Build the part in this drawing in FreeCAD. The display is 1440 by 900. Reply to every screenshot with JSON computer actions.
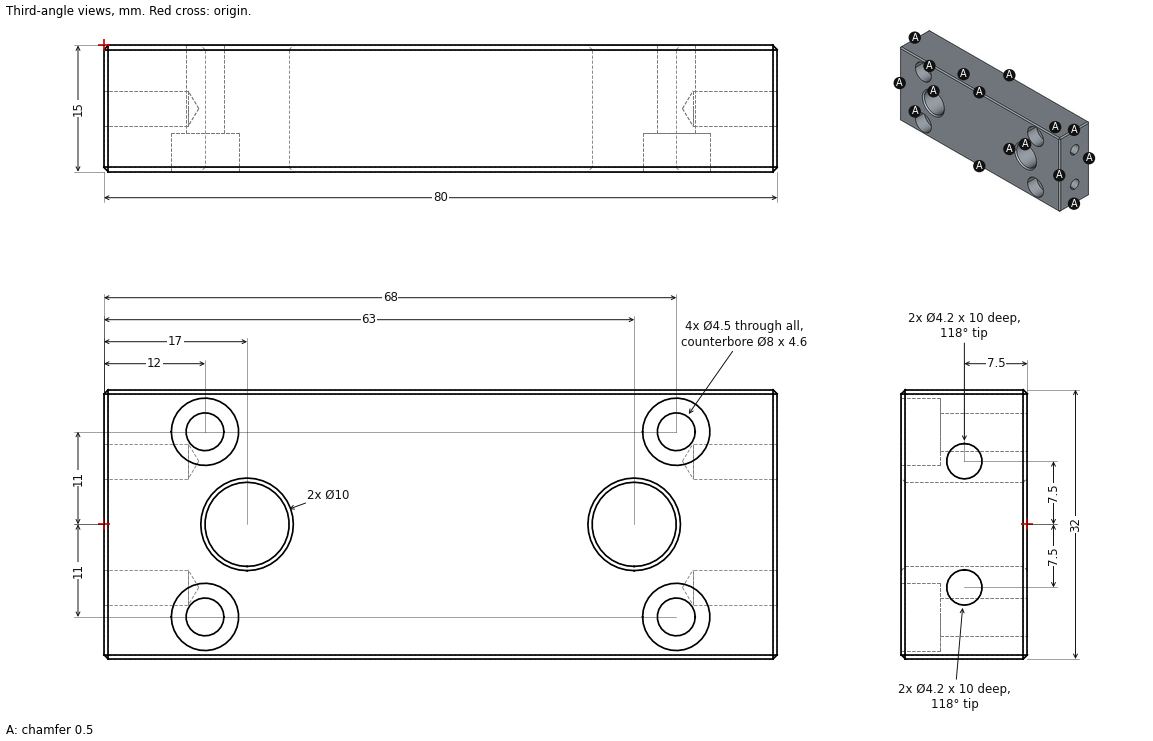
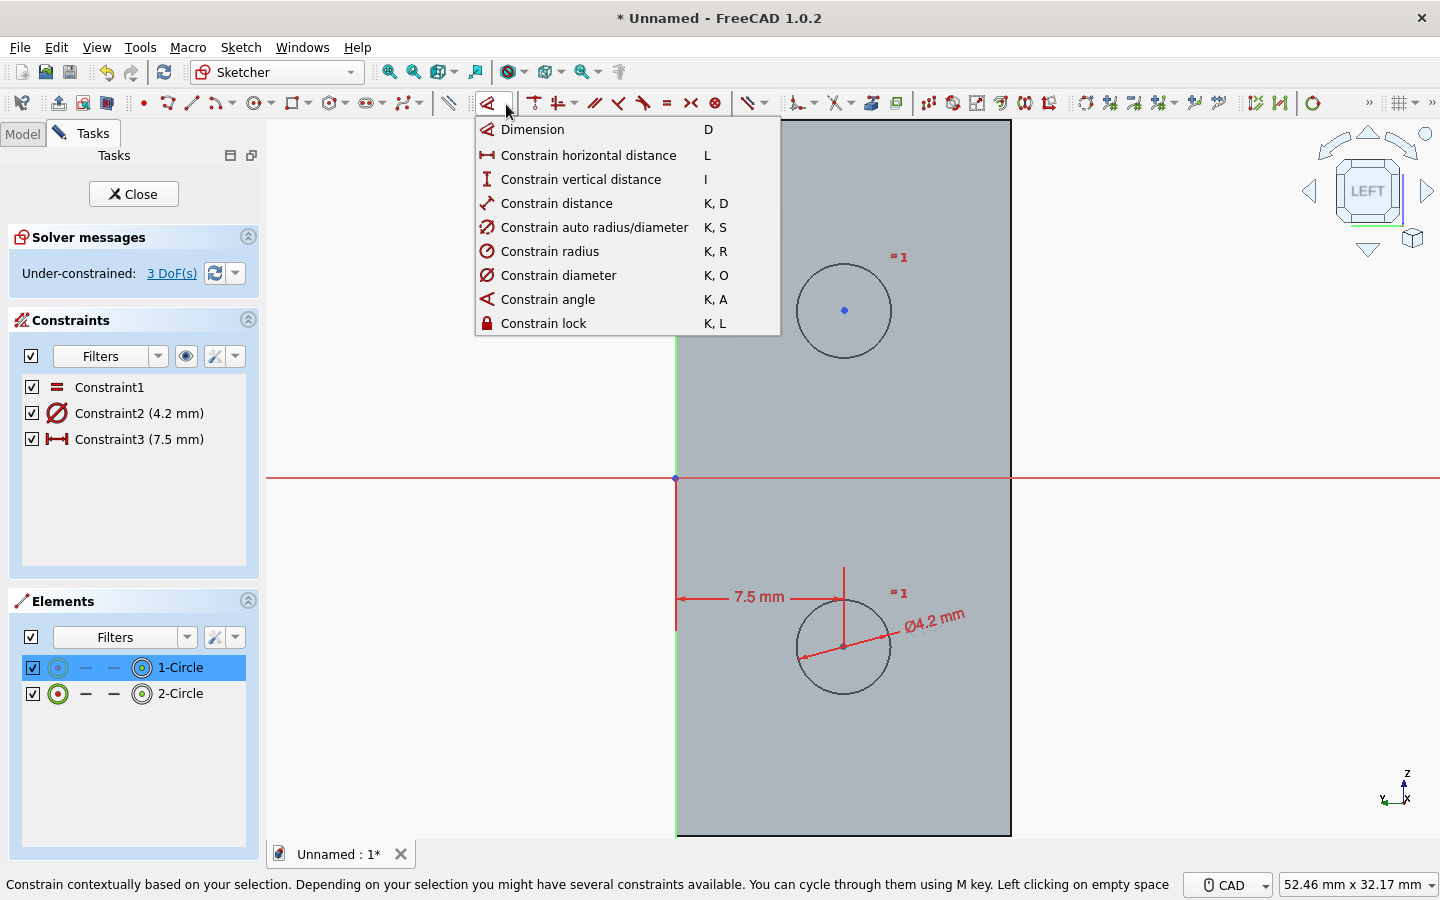
{"action": "left_click", "coordinate": [628, 179]}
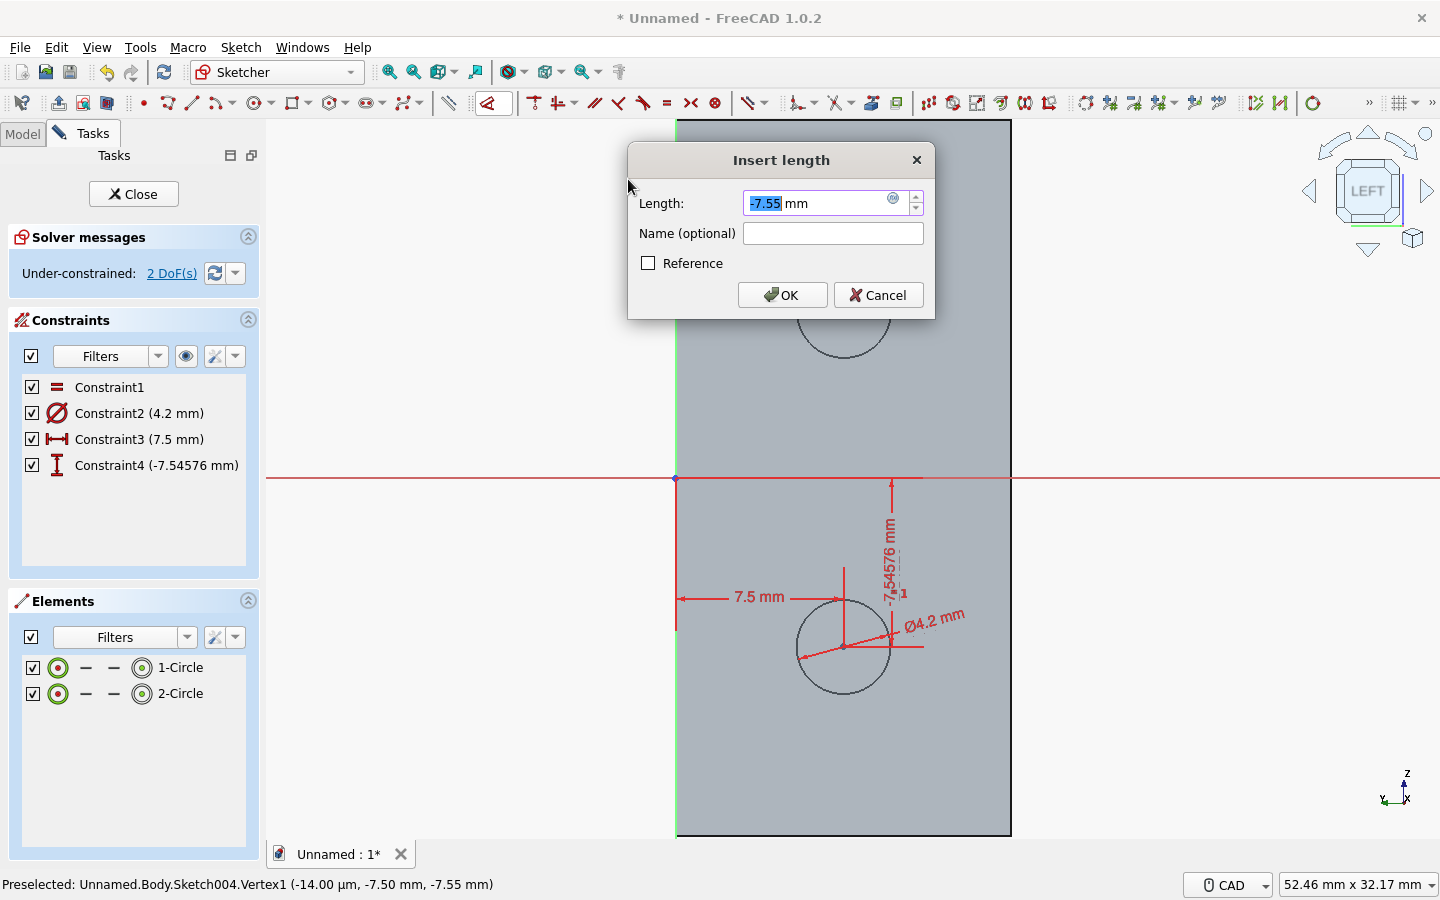
{"action": "type", "text": "-7.5"}
{"action": "key", "text": "Return"}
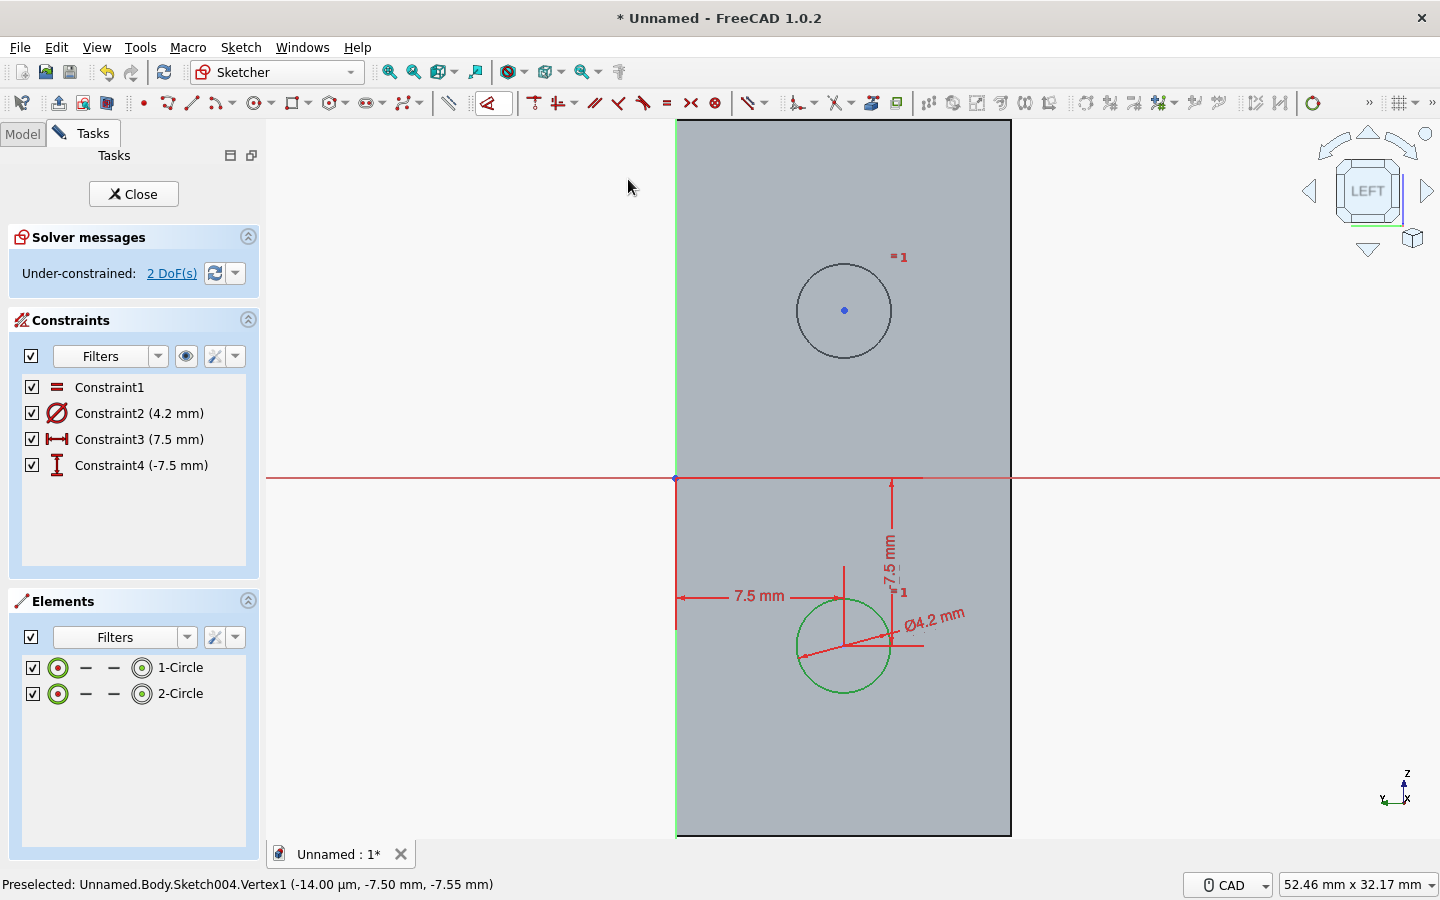
{"action": "left_click", "coordinate": [844, 311]}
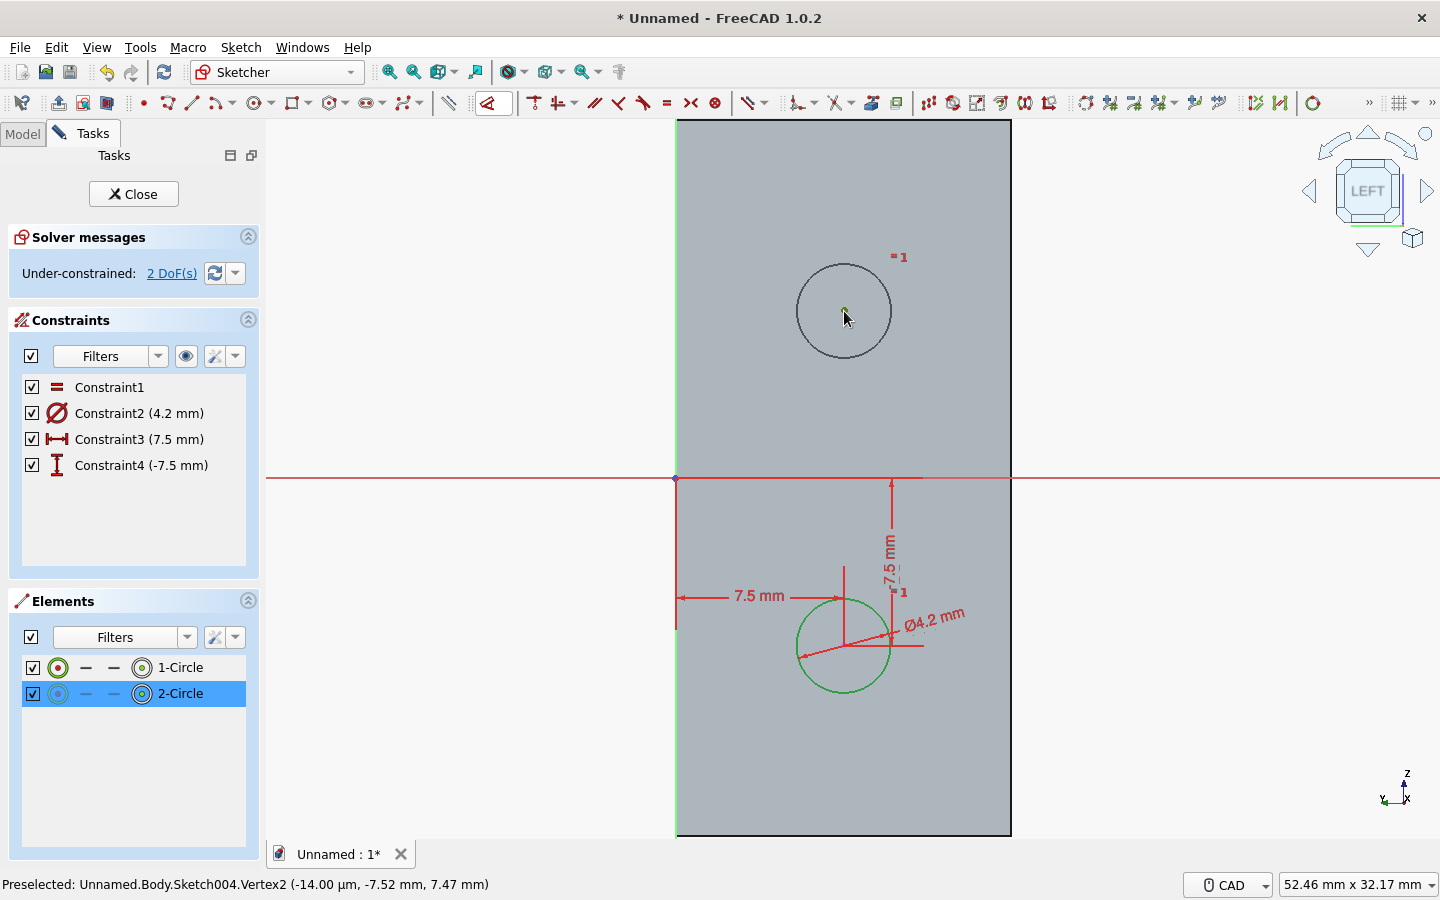
{"action": "left_click", "coordinate": [506, 104]}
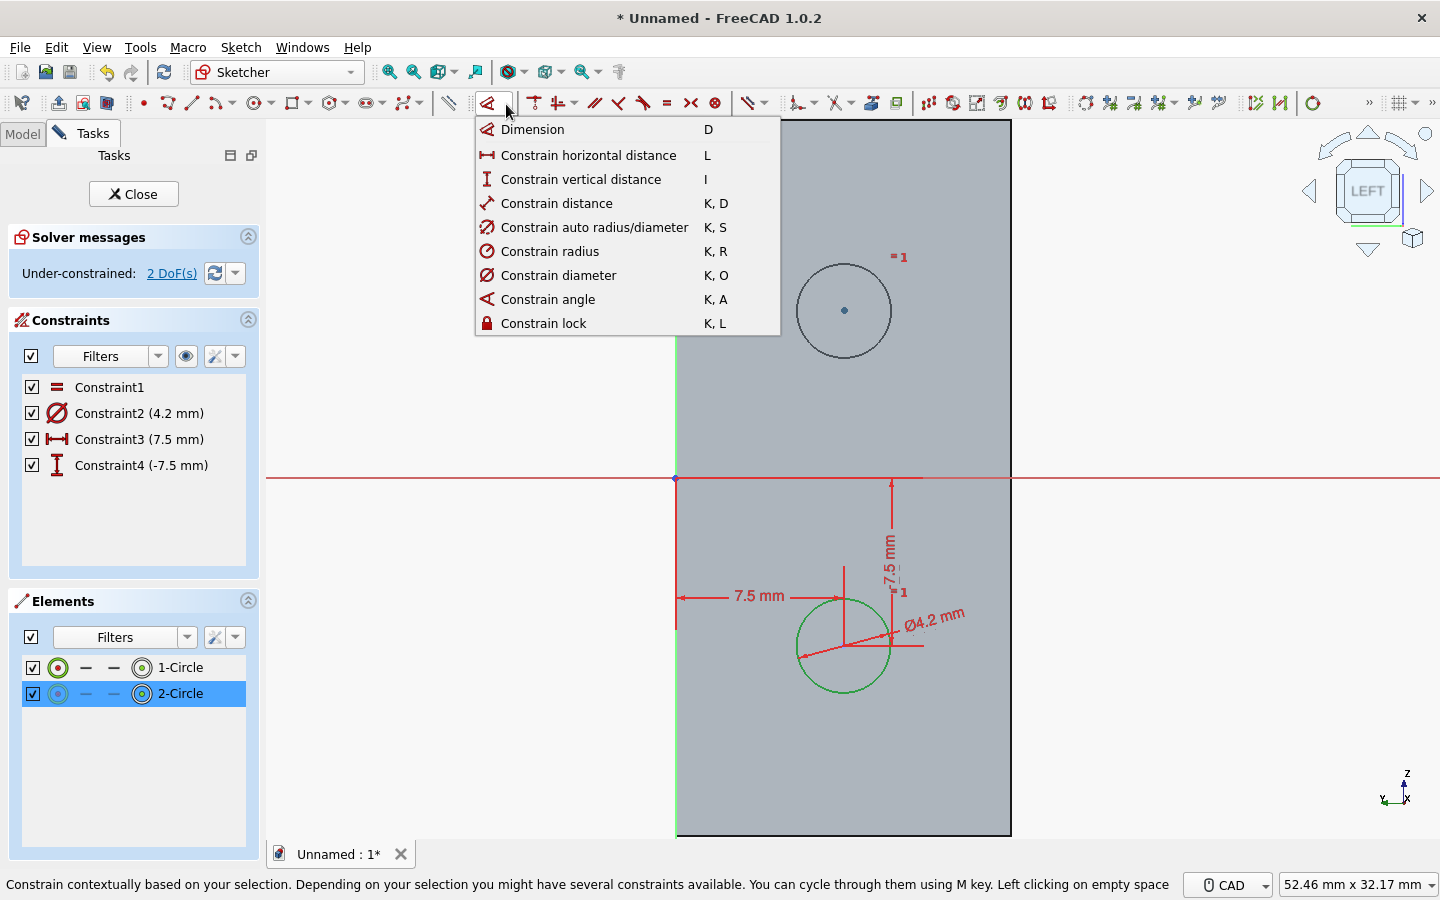
{"action": "left_click", "coordinate": [628, 155]}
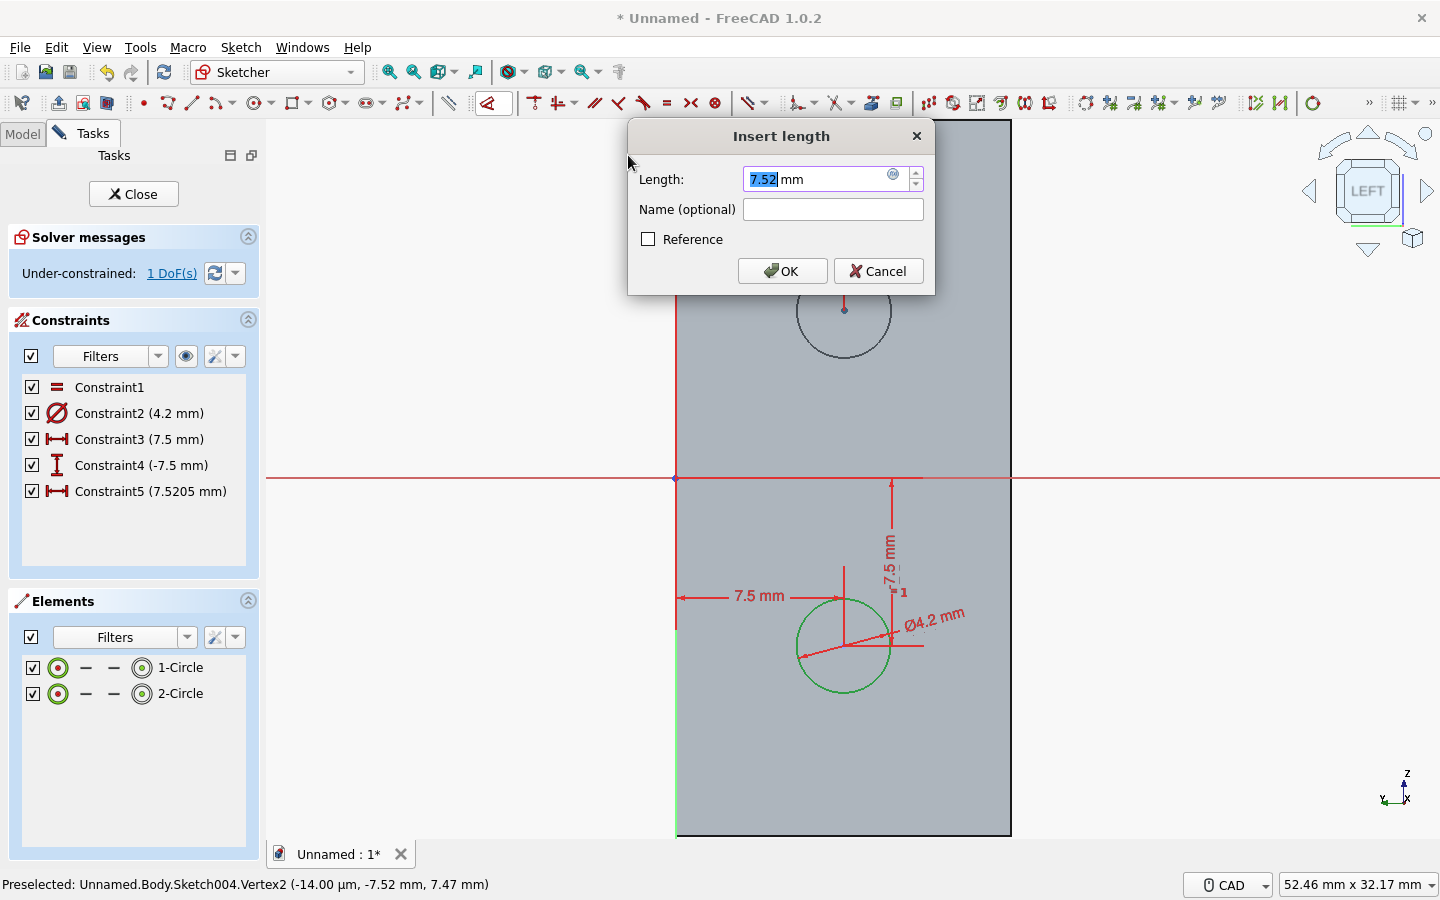
{"action": "type", "text": "7.5"}
{"action": "key", "text": "Return"}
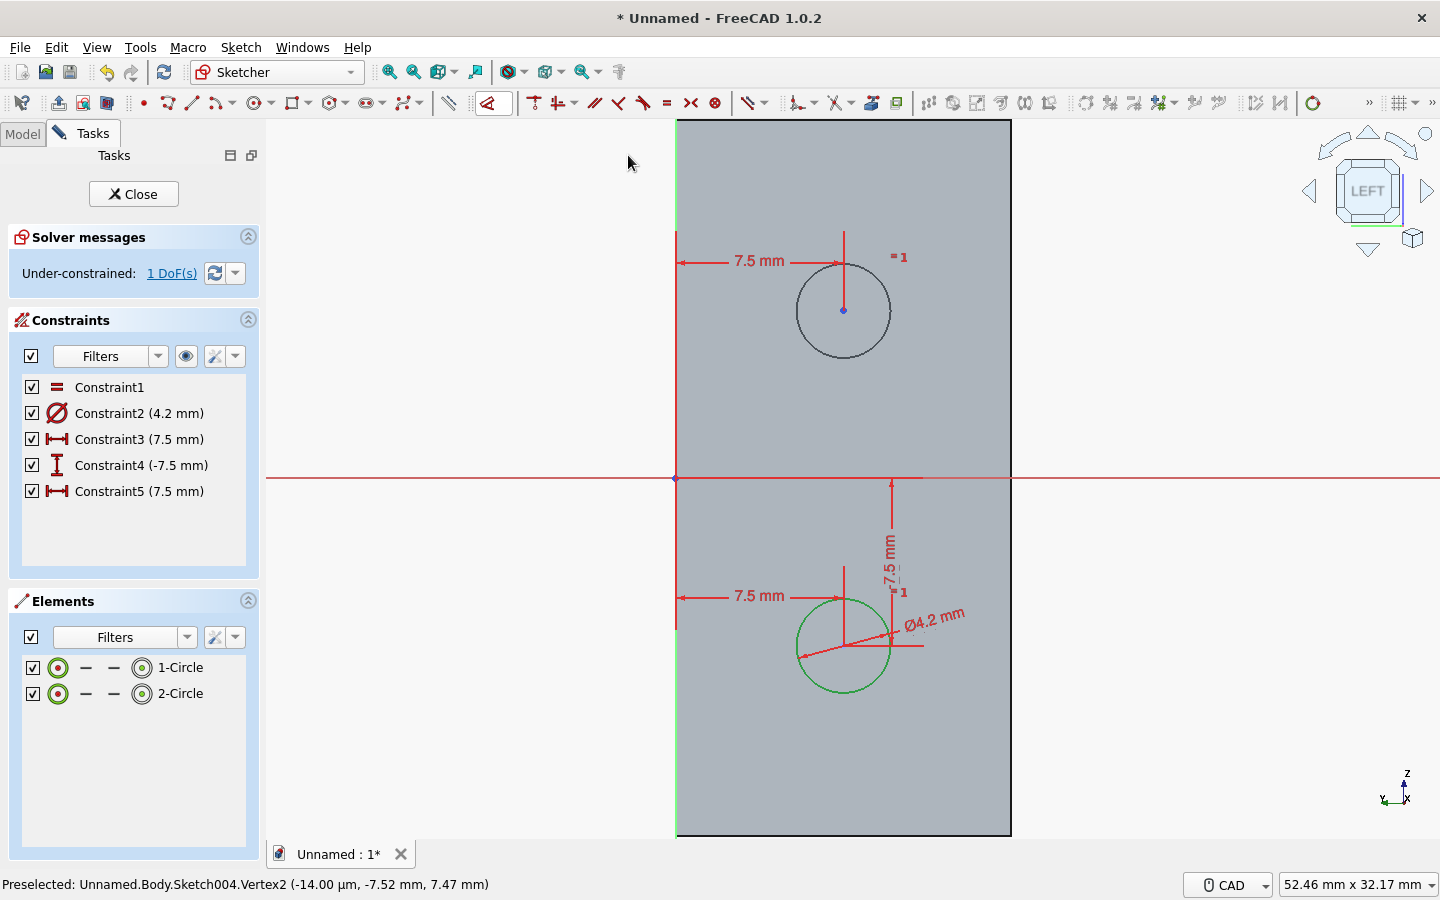
{"action": "left_click", "coordinate": [844, 311]}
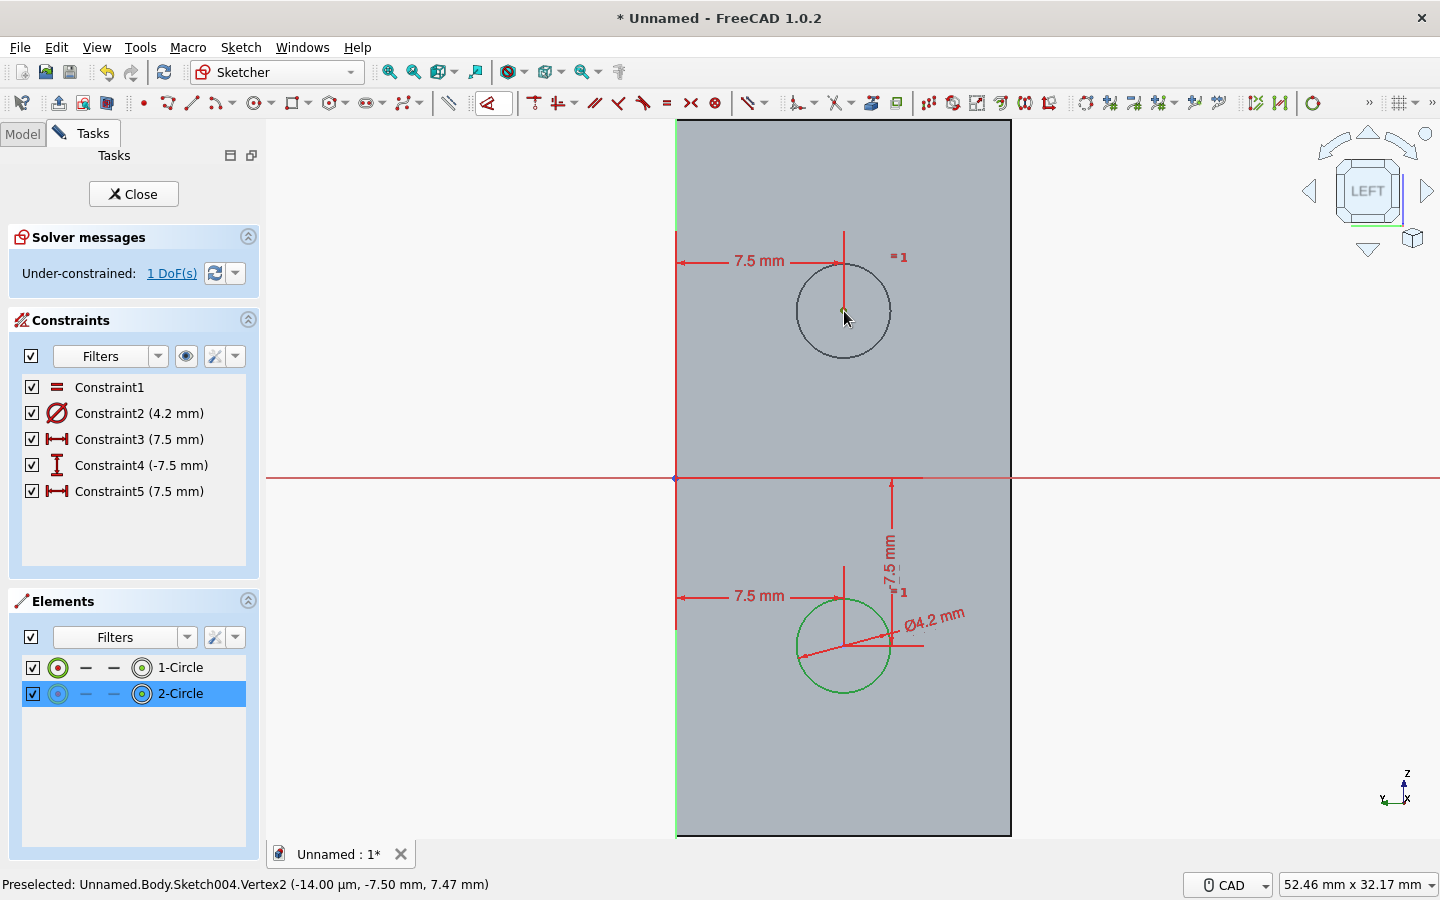
{"action": "left_click", "coordinate": [506, 104]}